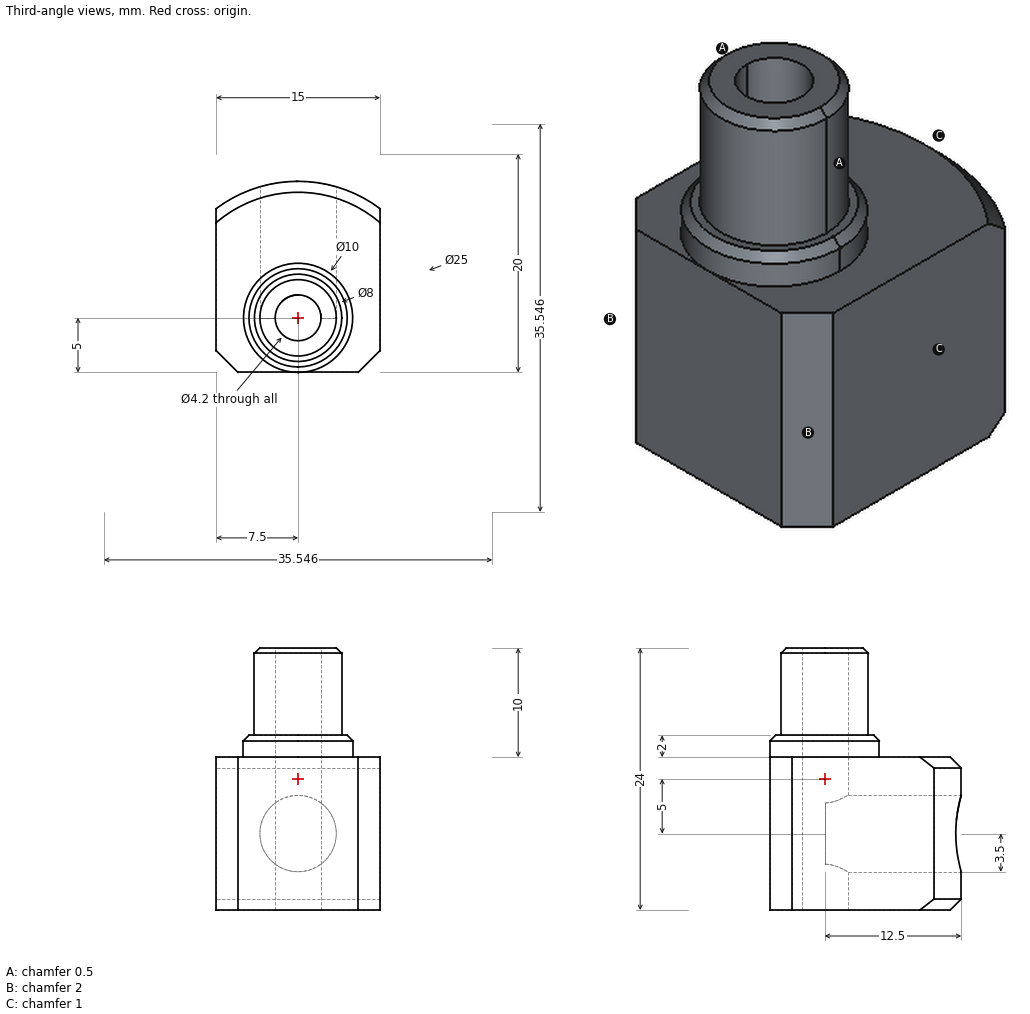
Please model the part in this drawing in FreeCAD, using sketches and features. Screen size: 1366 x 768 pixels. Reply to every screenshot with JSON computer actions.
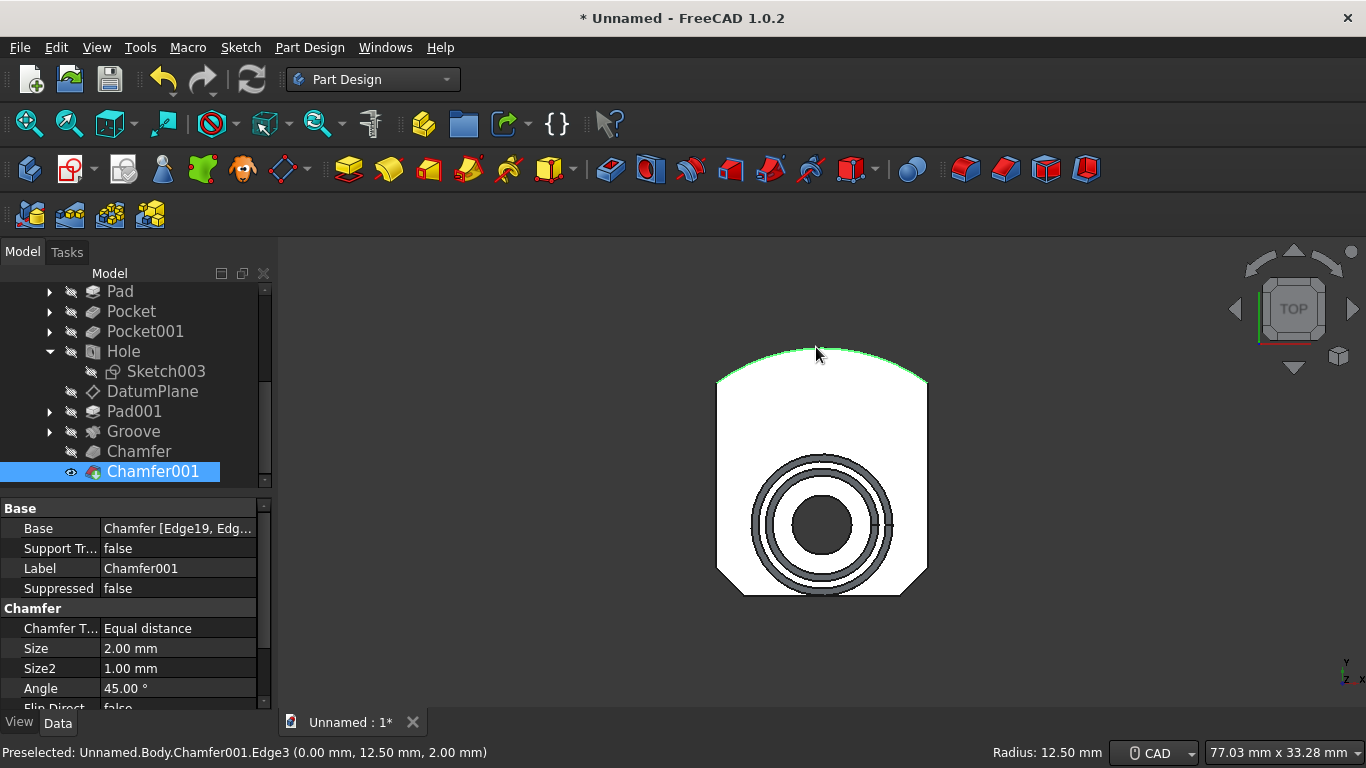
{"action": "key", "text": "1"}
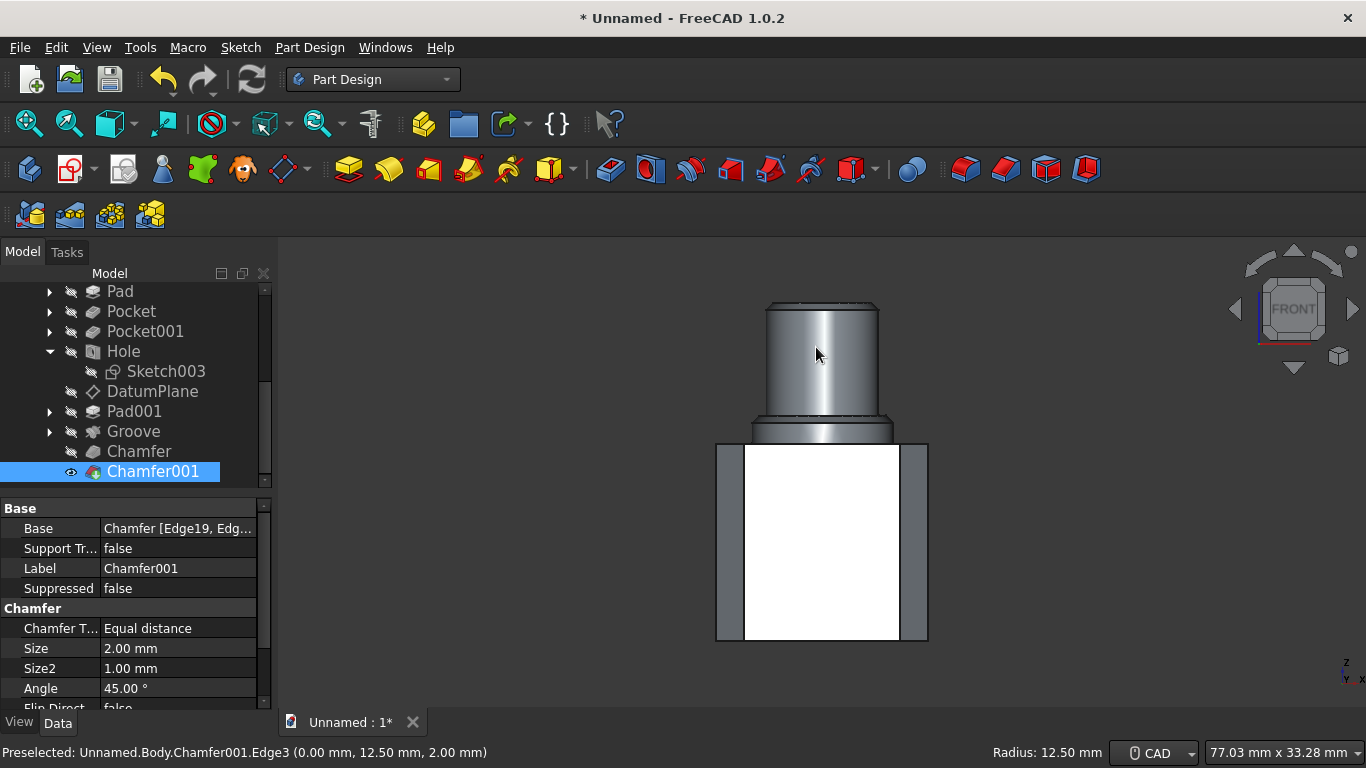
{"action": "key", "text": "3"}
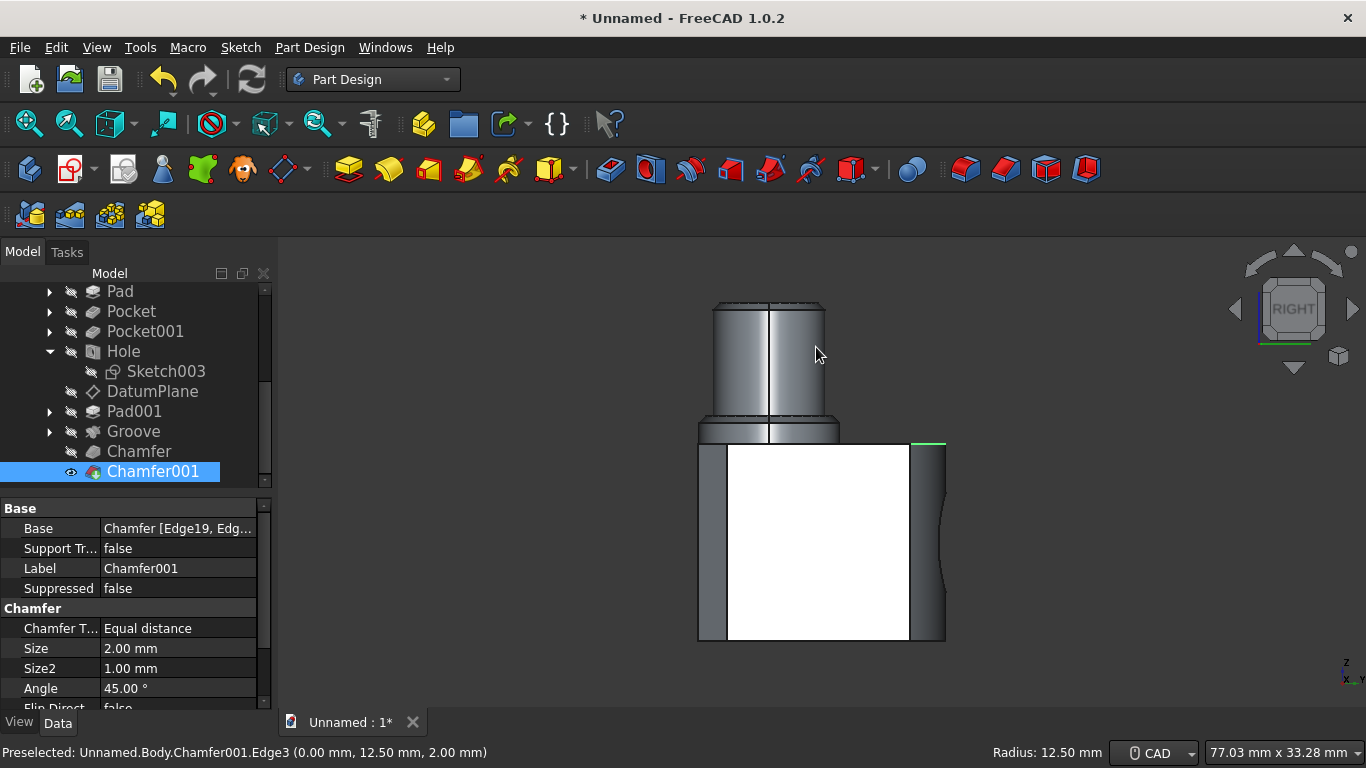
{"action": "left_click", "coordinate": [933, 640], "text": "ctrl"}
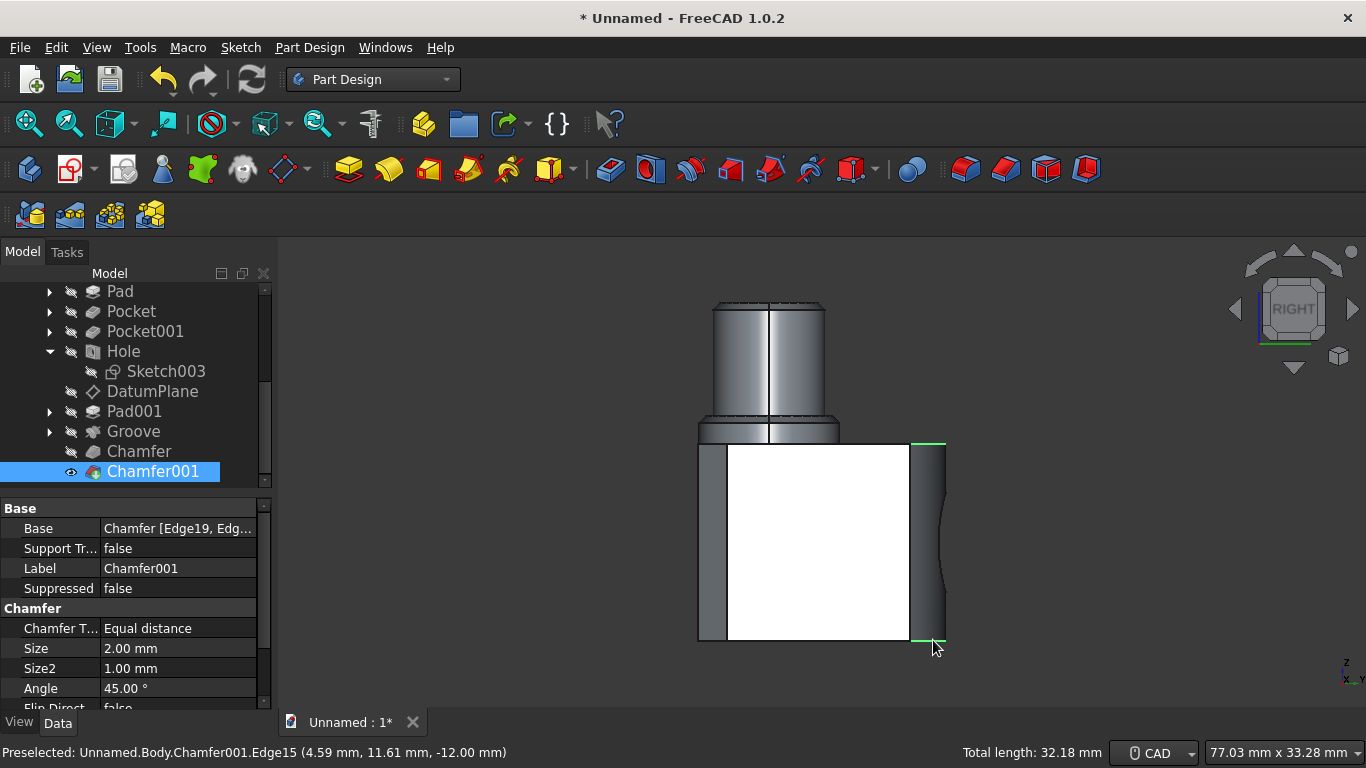
{"action": "left_click", "coordinate": [1006, 170]}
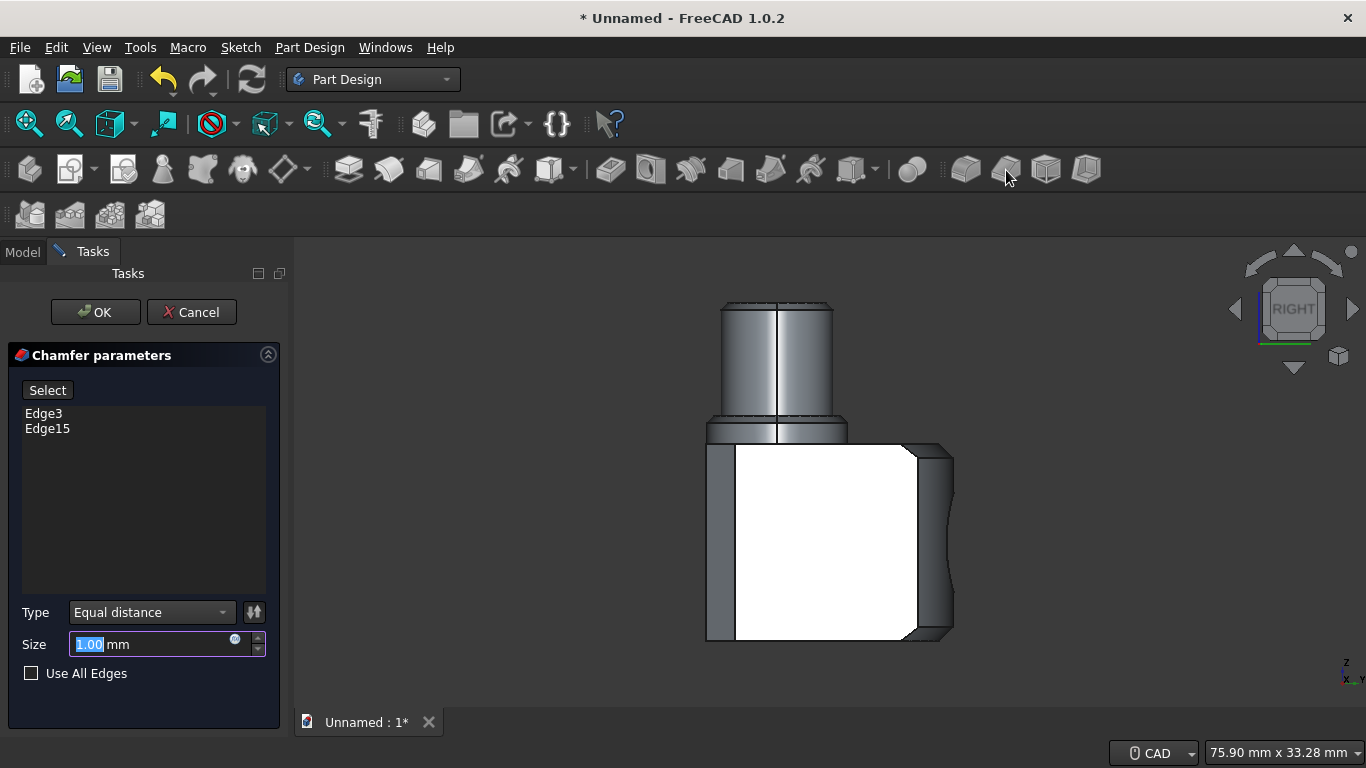
{"action": "type", "text": "1"}
{"action": "key", "text": "Tab"}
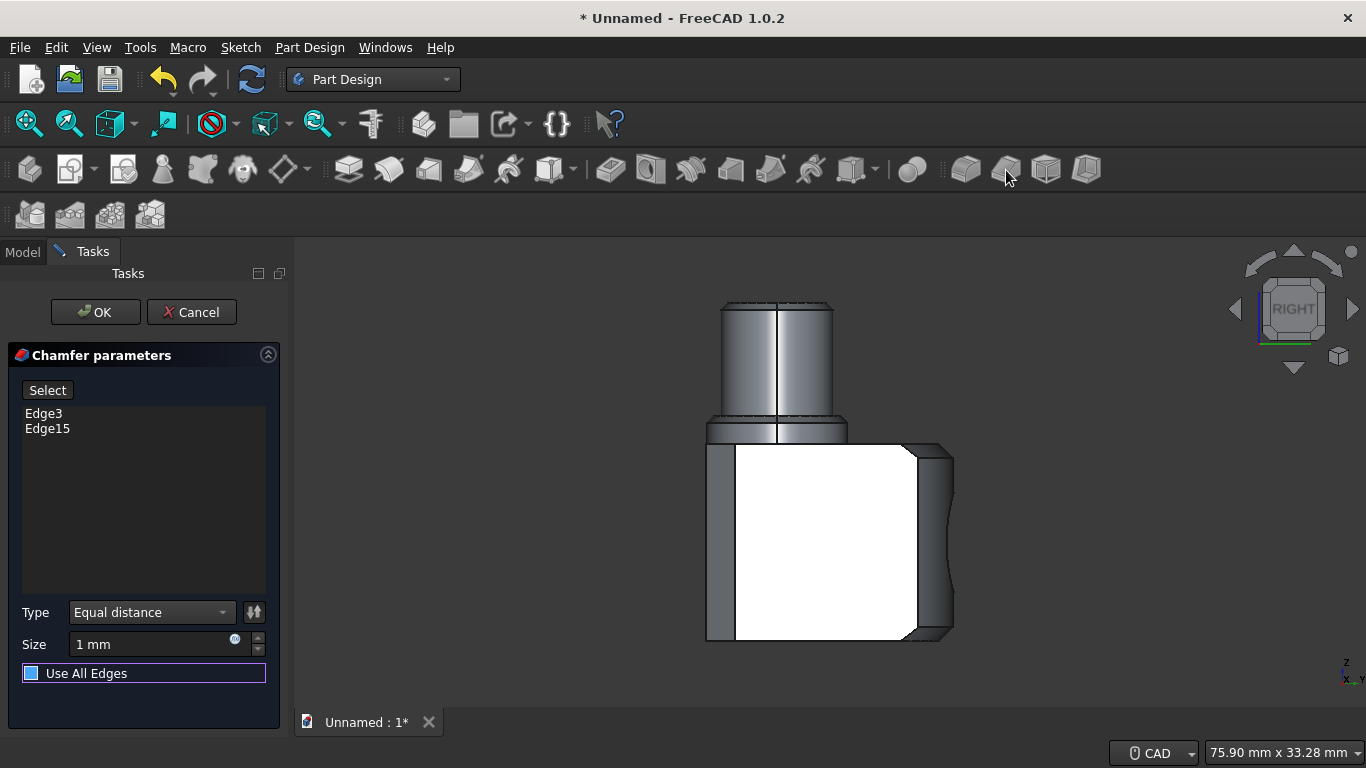
{"action": "left_click", "coordinate": [96, 312]}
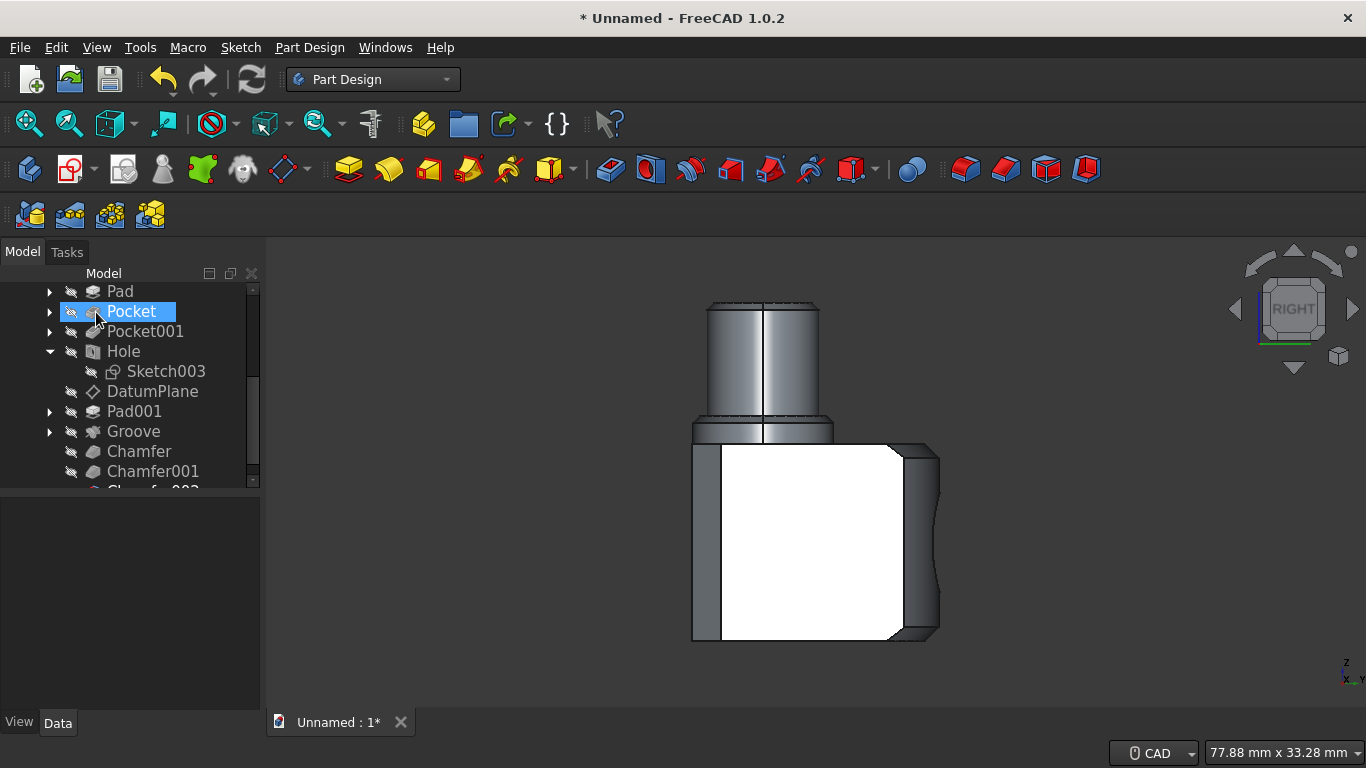
{"action": "key", "text": "0"}